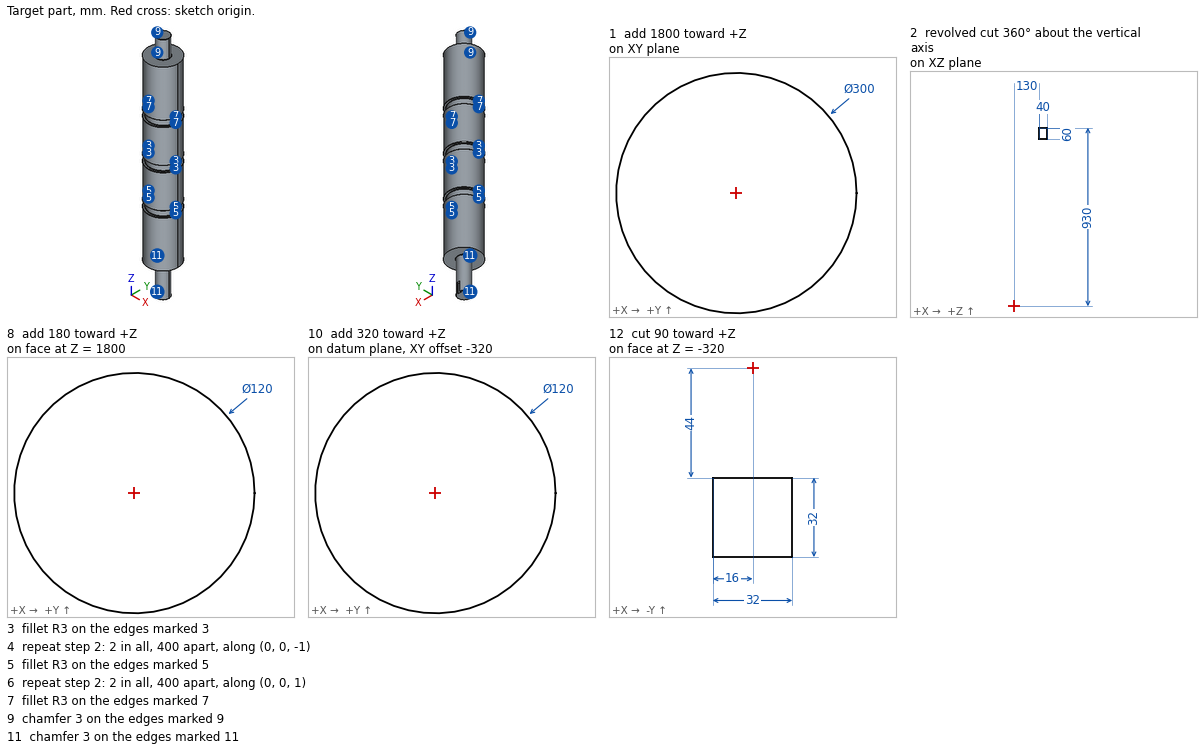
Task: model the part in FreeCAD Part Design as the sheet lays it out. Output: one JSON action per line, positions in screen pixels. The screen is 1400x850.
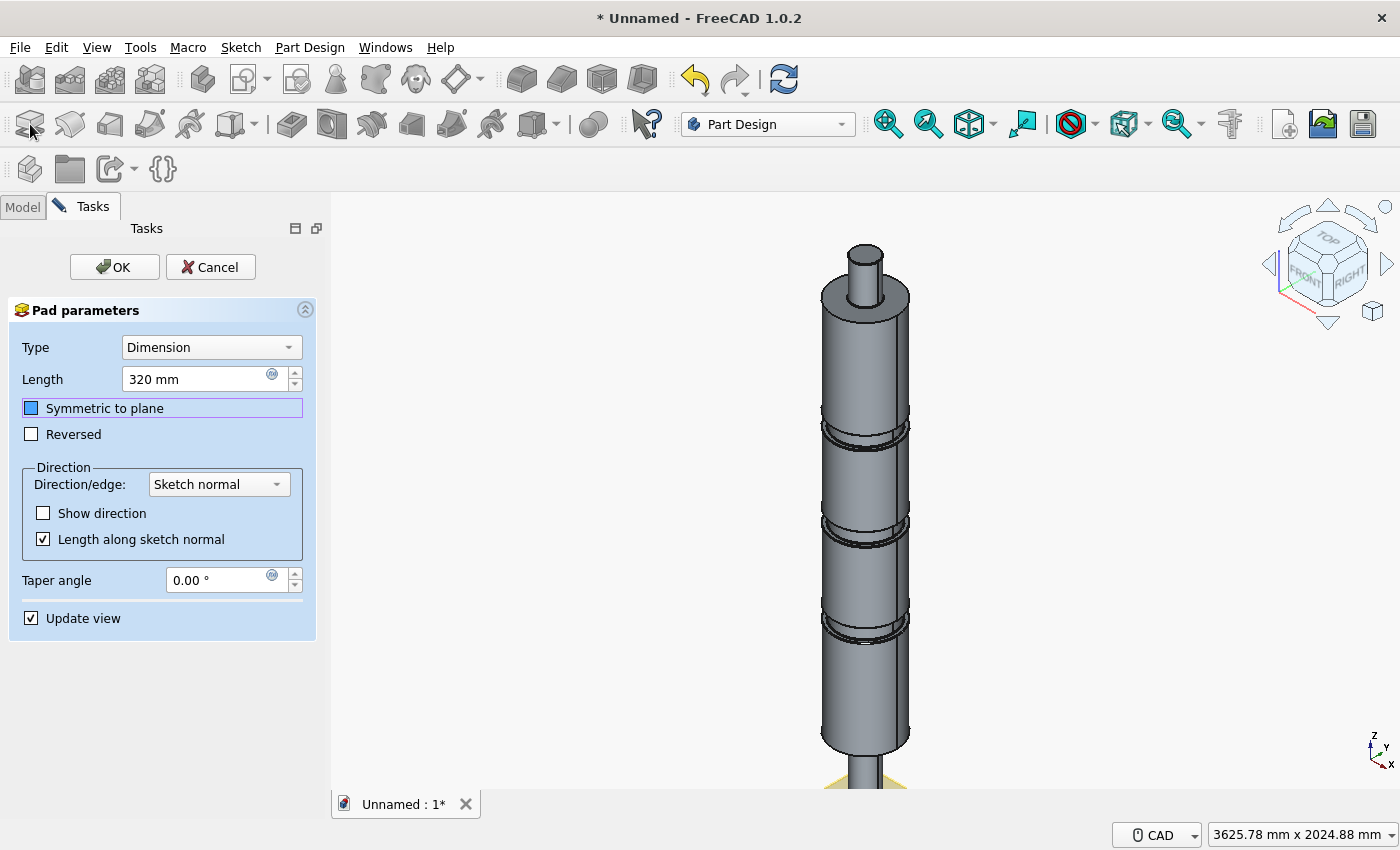
{"action": "left_click", "coordinate": [115, 267]}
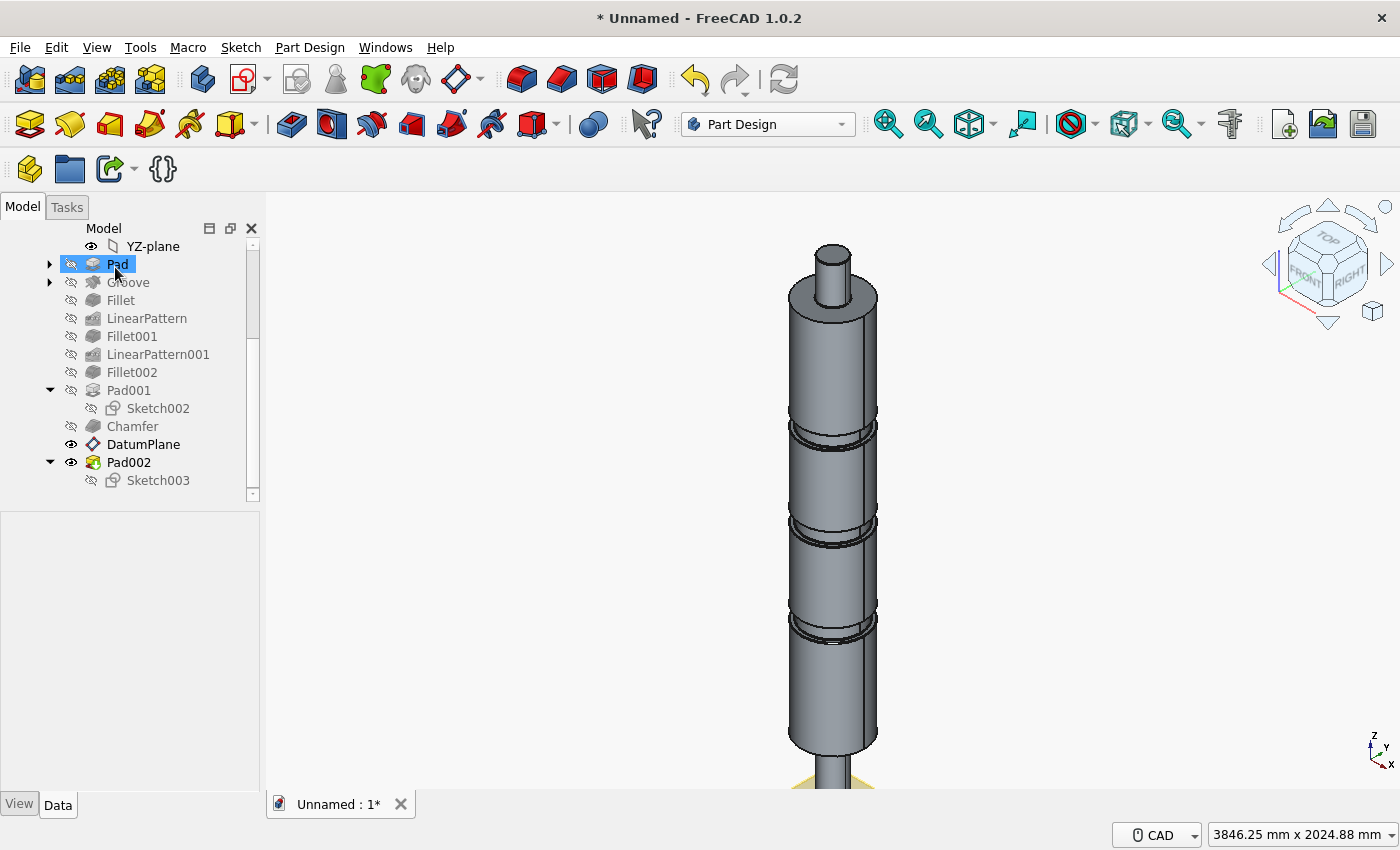
{"action": "left_click", "coordinate": [116, 444]}
{"action": "key", "text": "space"}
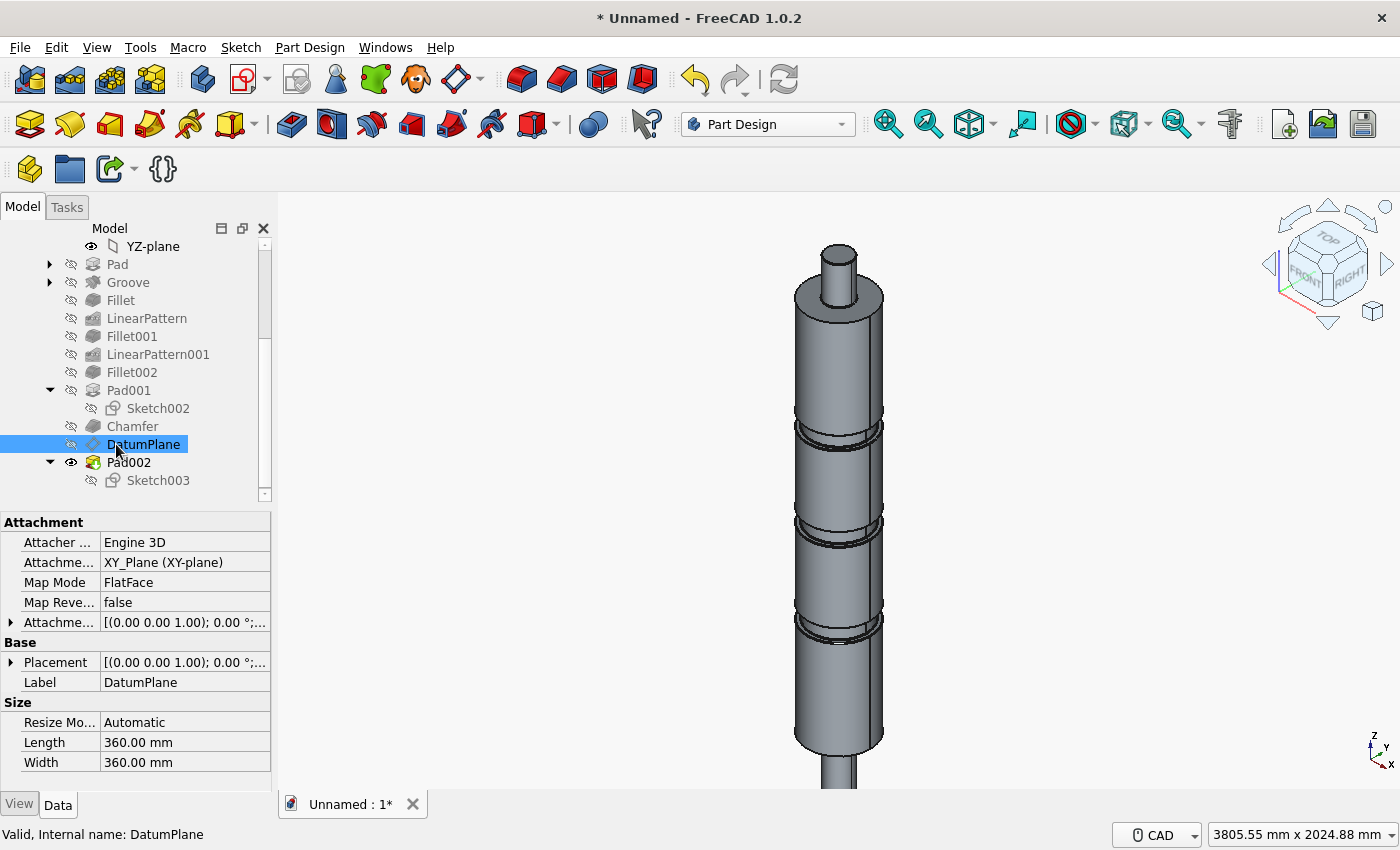
{"action": "left_click", "coordinate": [890, 124]}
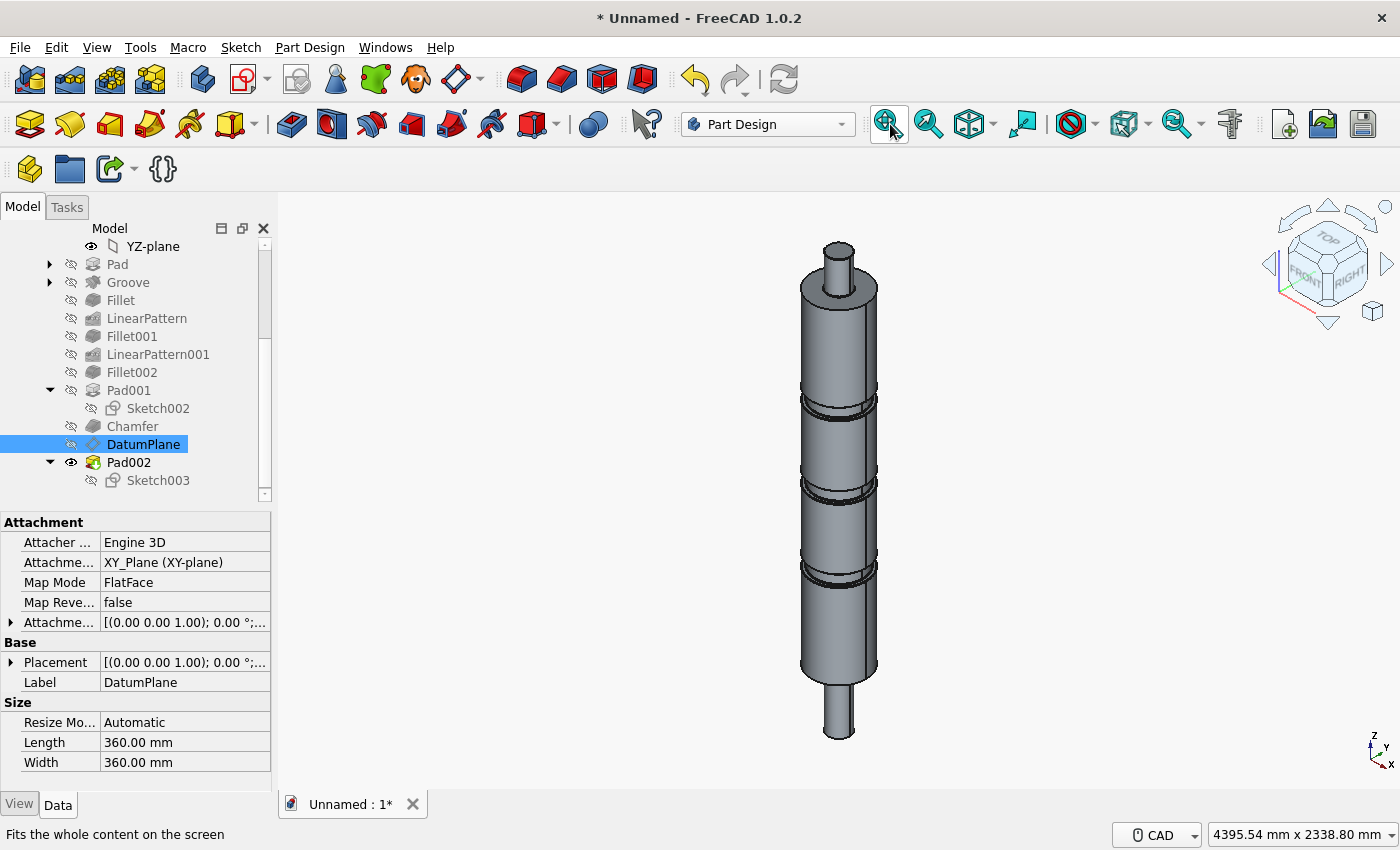
{"action": "left_click", "coordinate": [825, 733]}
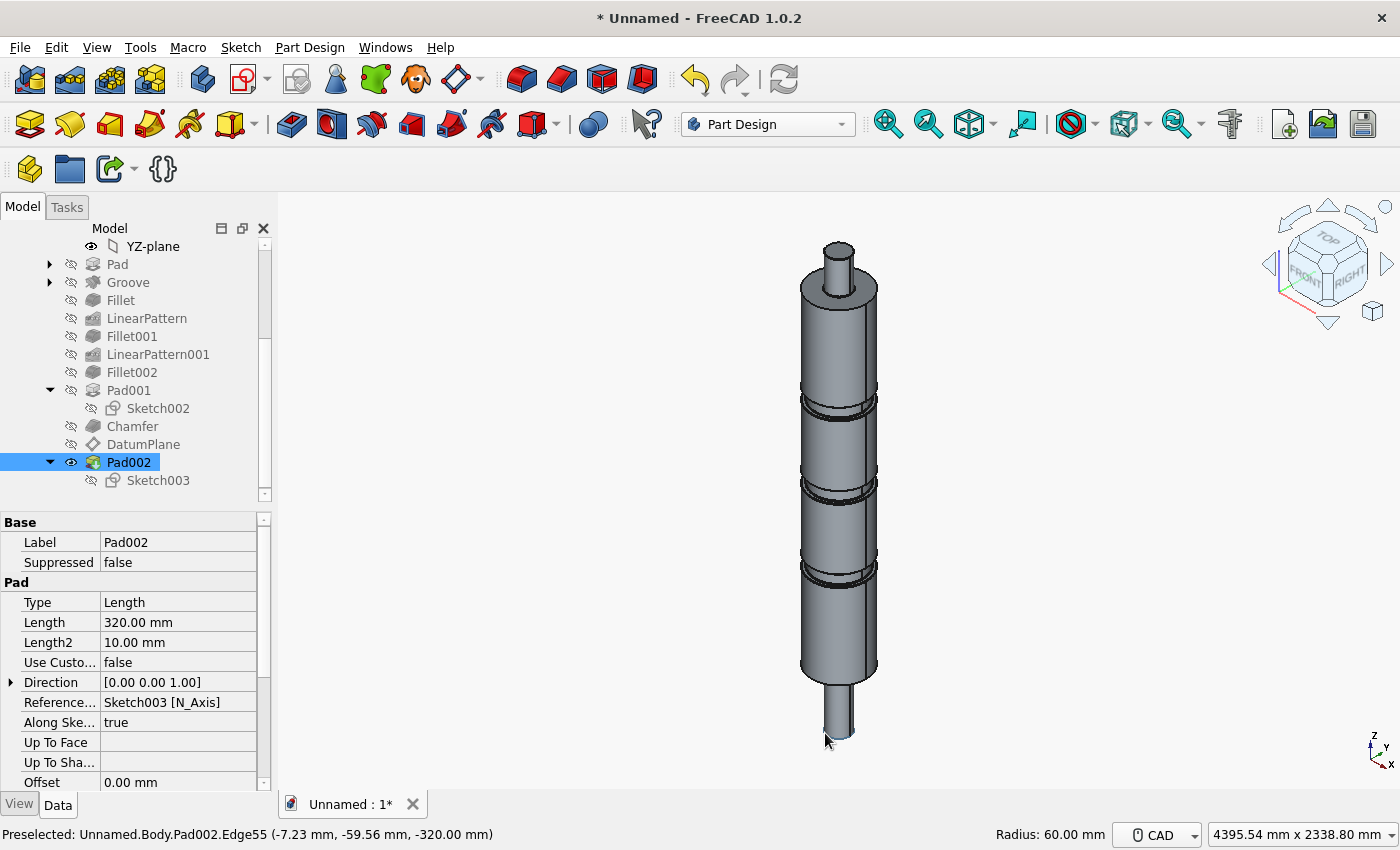
{"action": "key", "text": "2"}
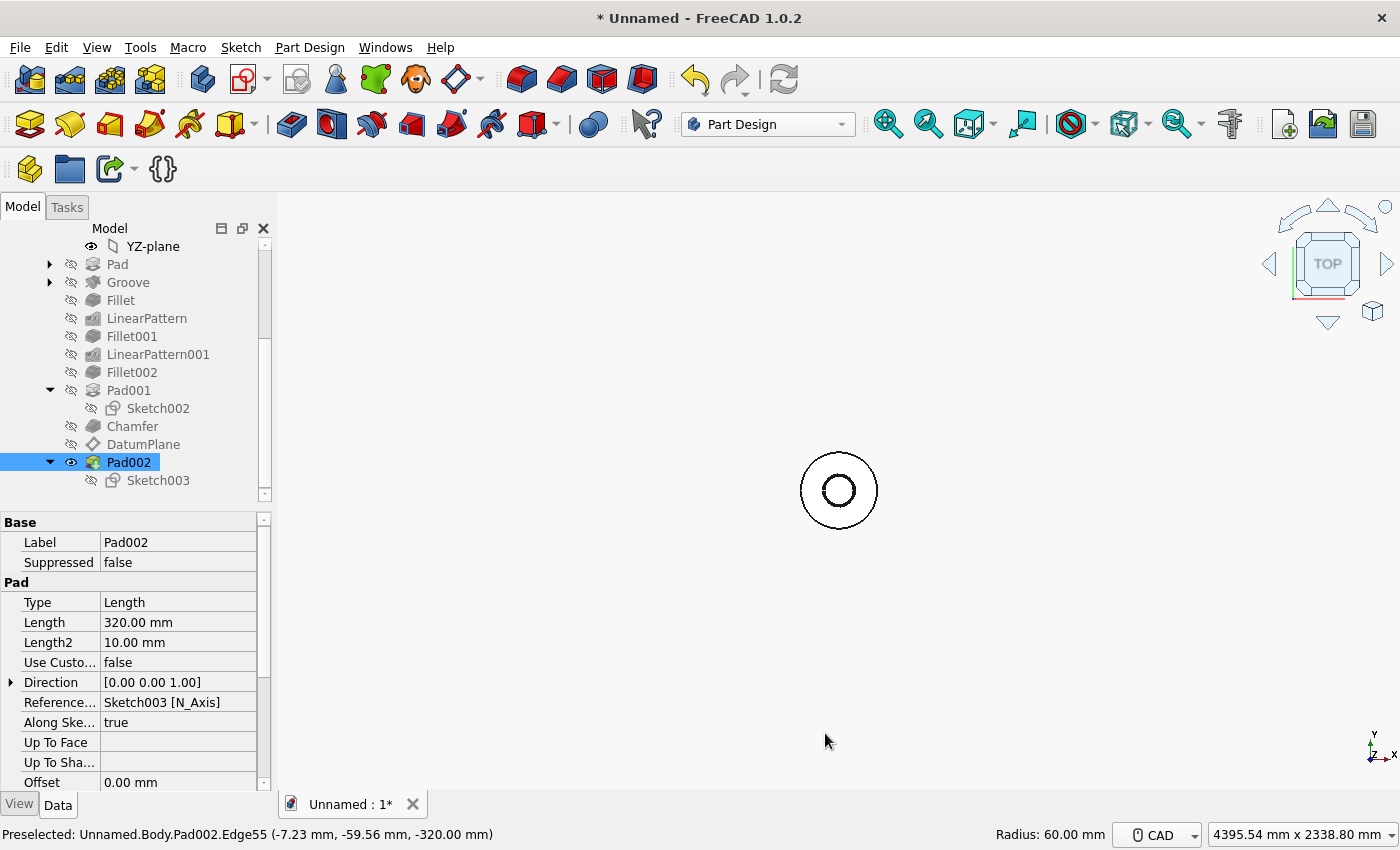
{"action": "left_click", "coordinate": [890, 124]}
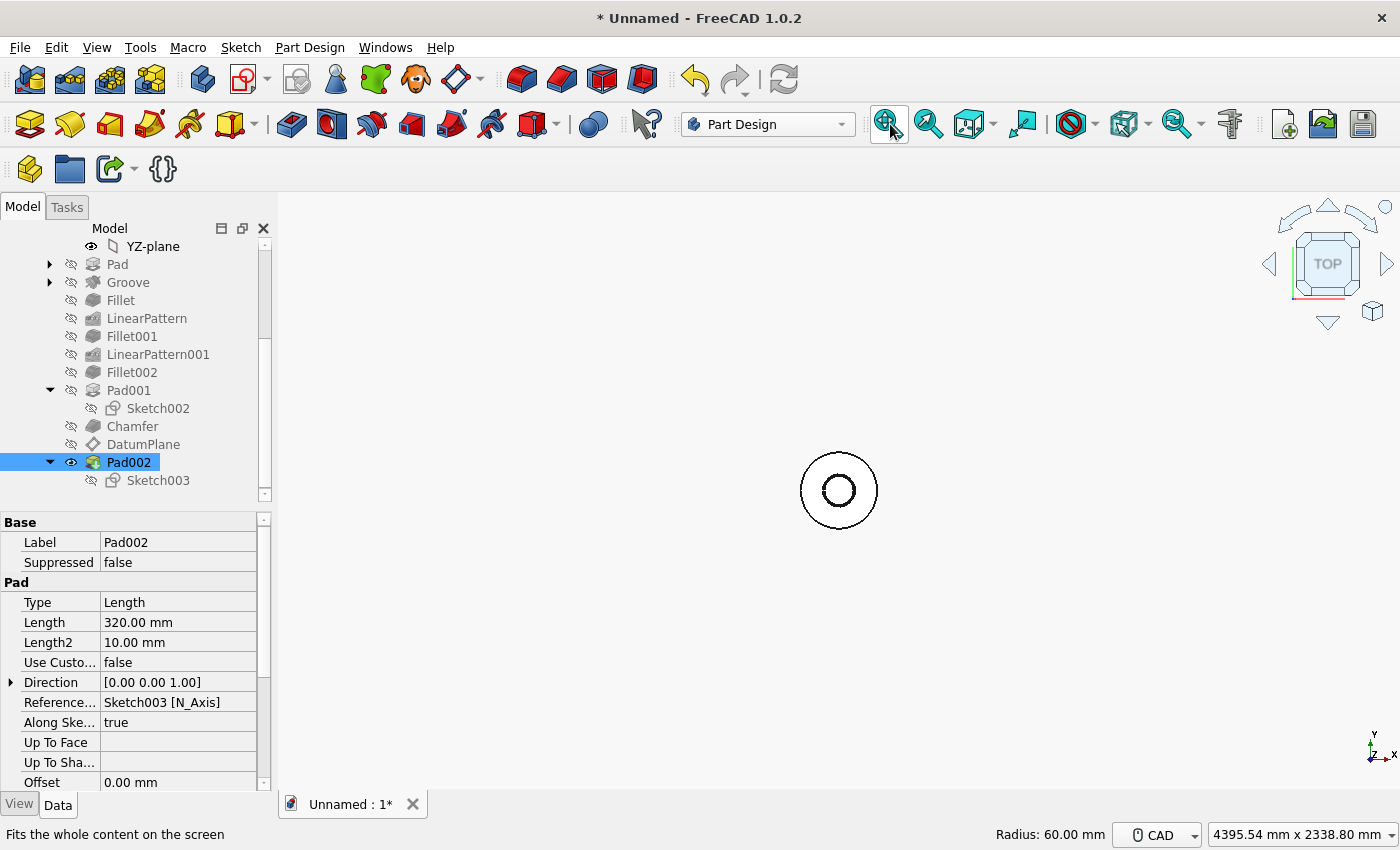
{"action": "key", "text": "0"}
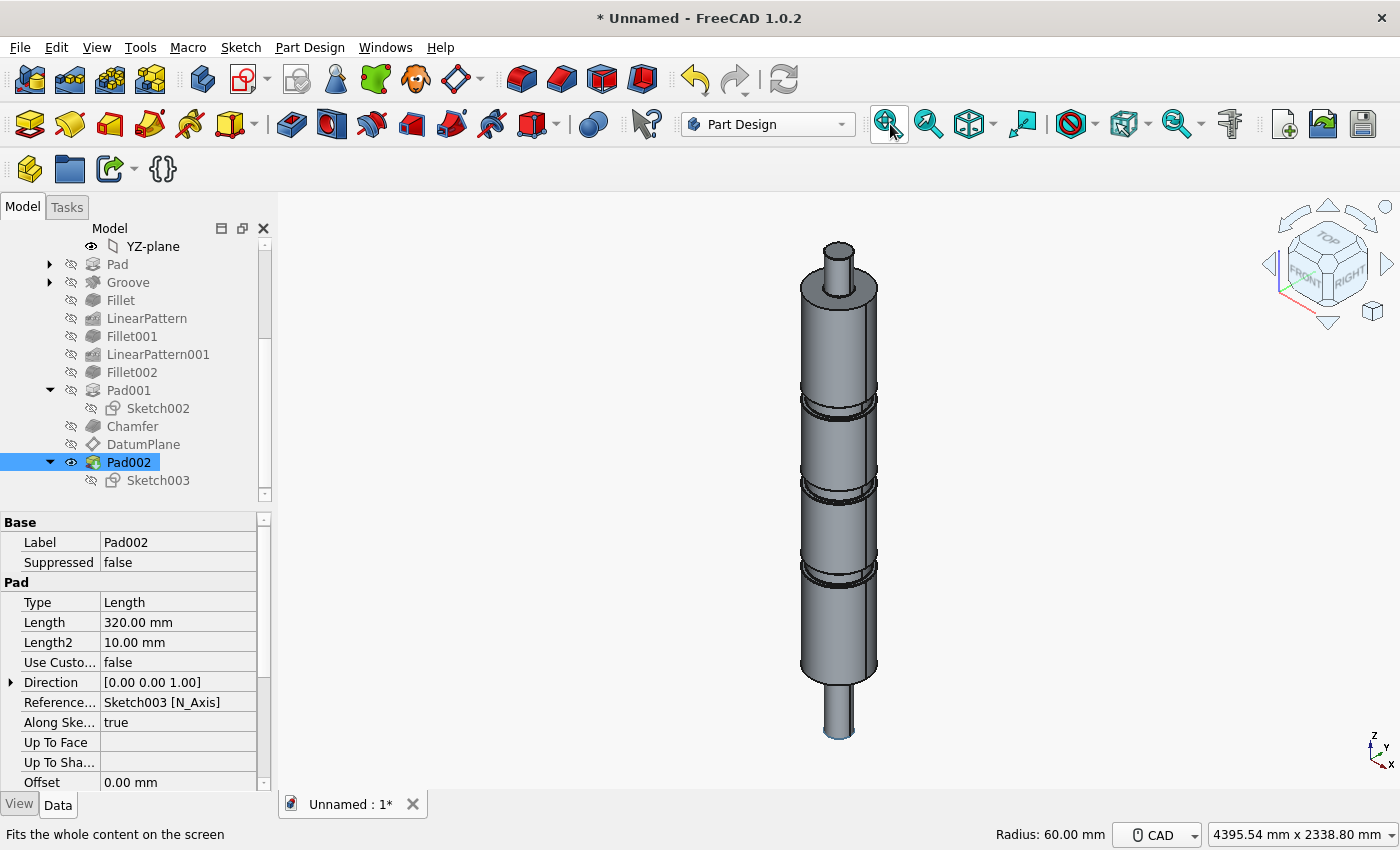
{"action": "key", "text": "1"}